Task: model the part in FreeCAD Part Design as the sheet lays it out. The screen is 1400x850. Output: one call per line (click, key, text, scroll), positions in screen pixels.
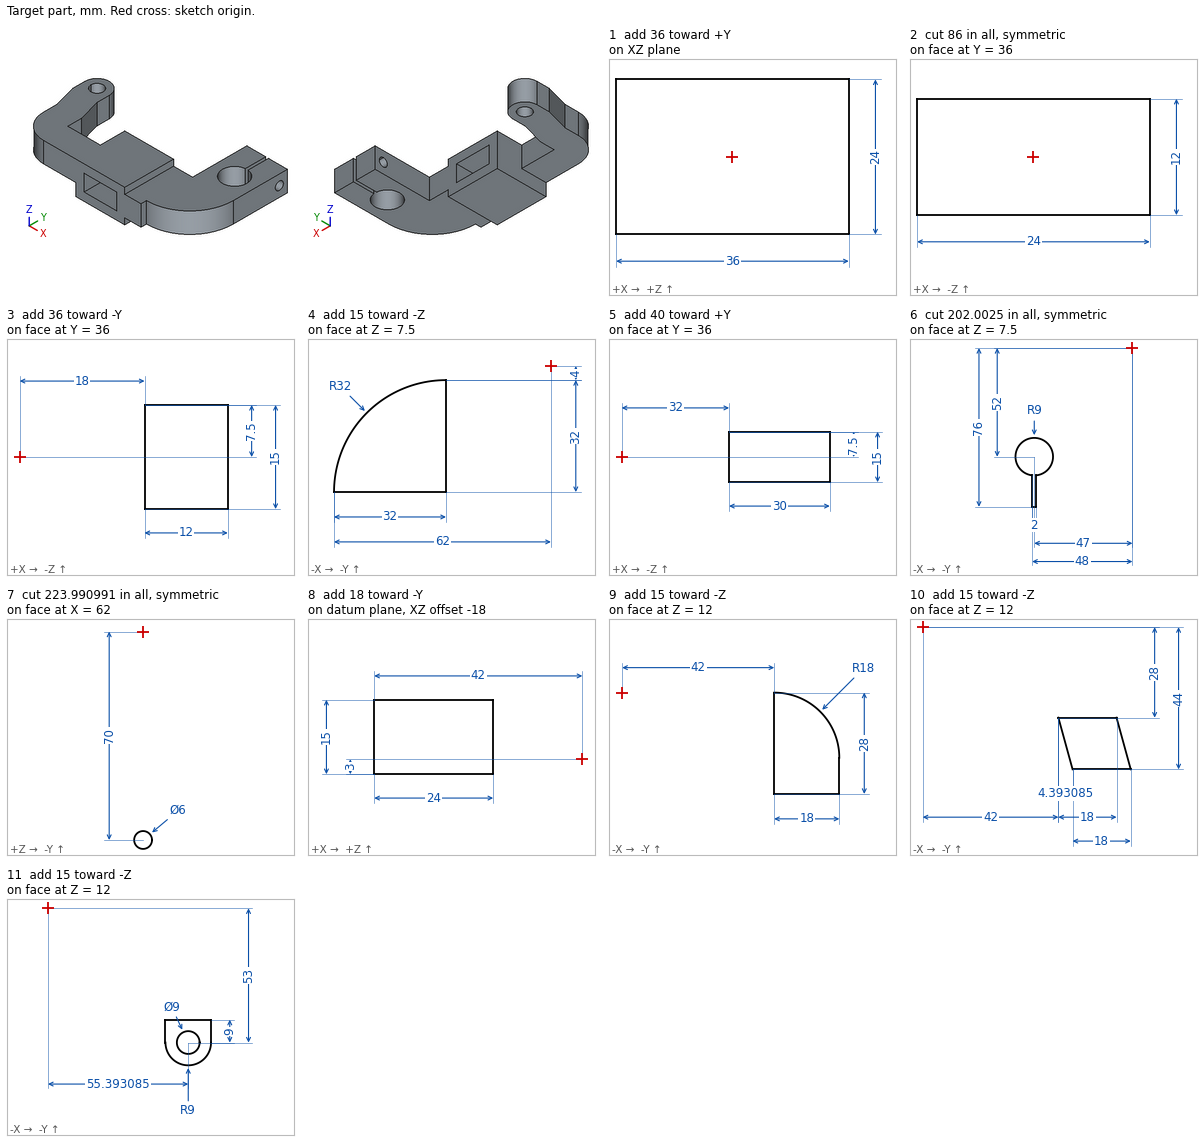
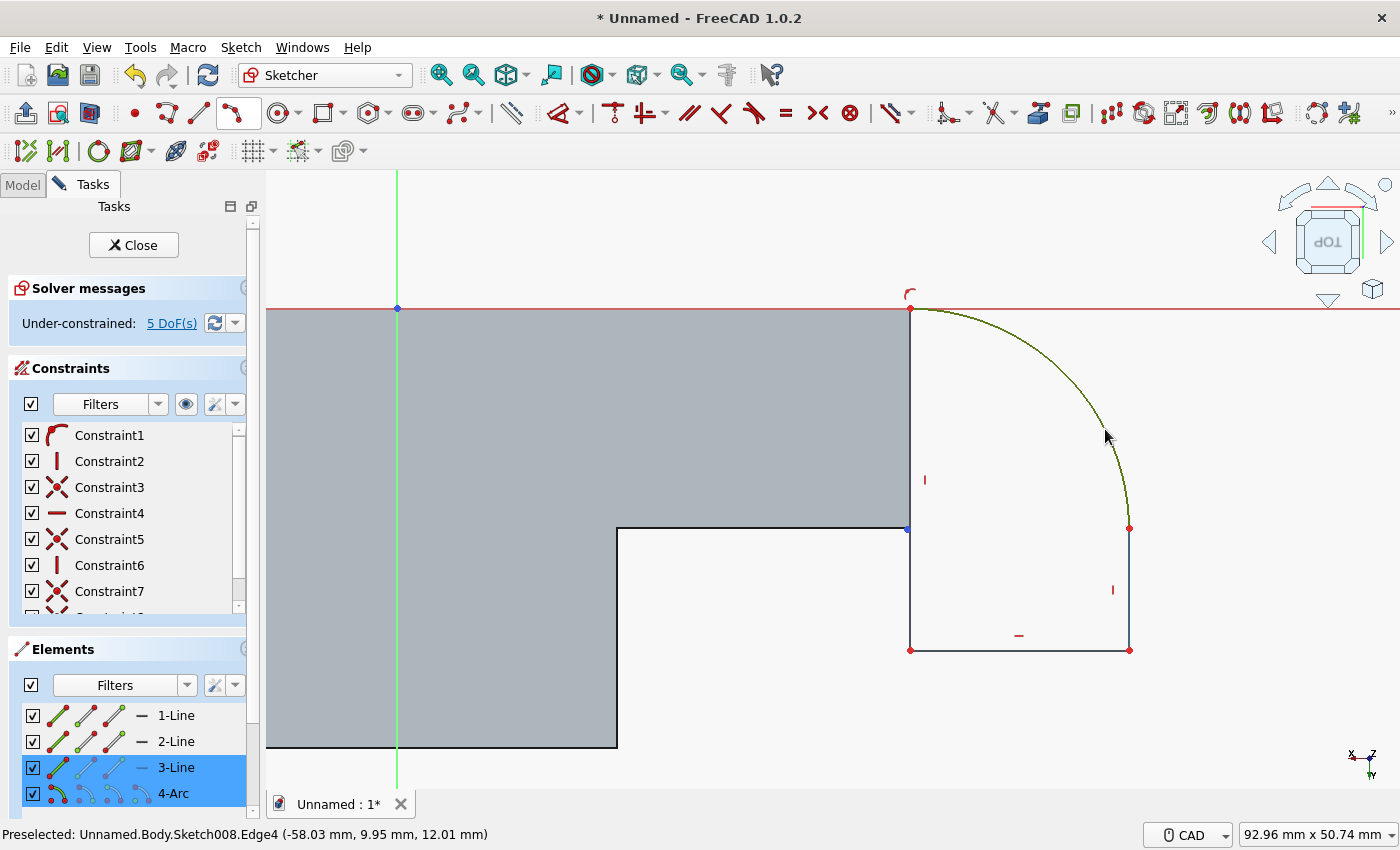
key(t)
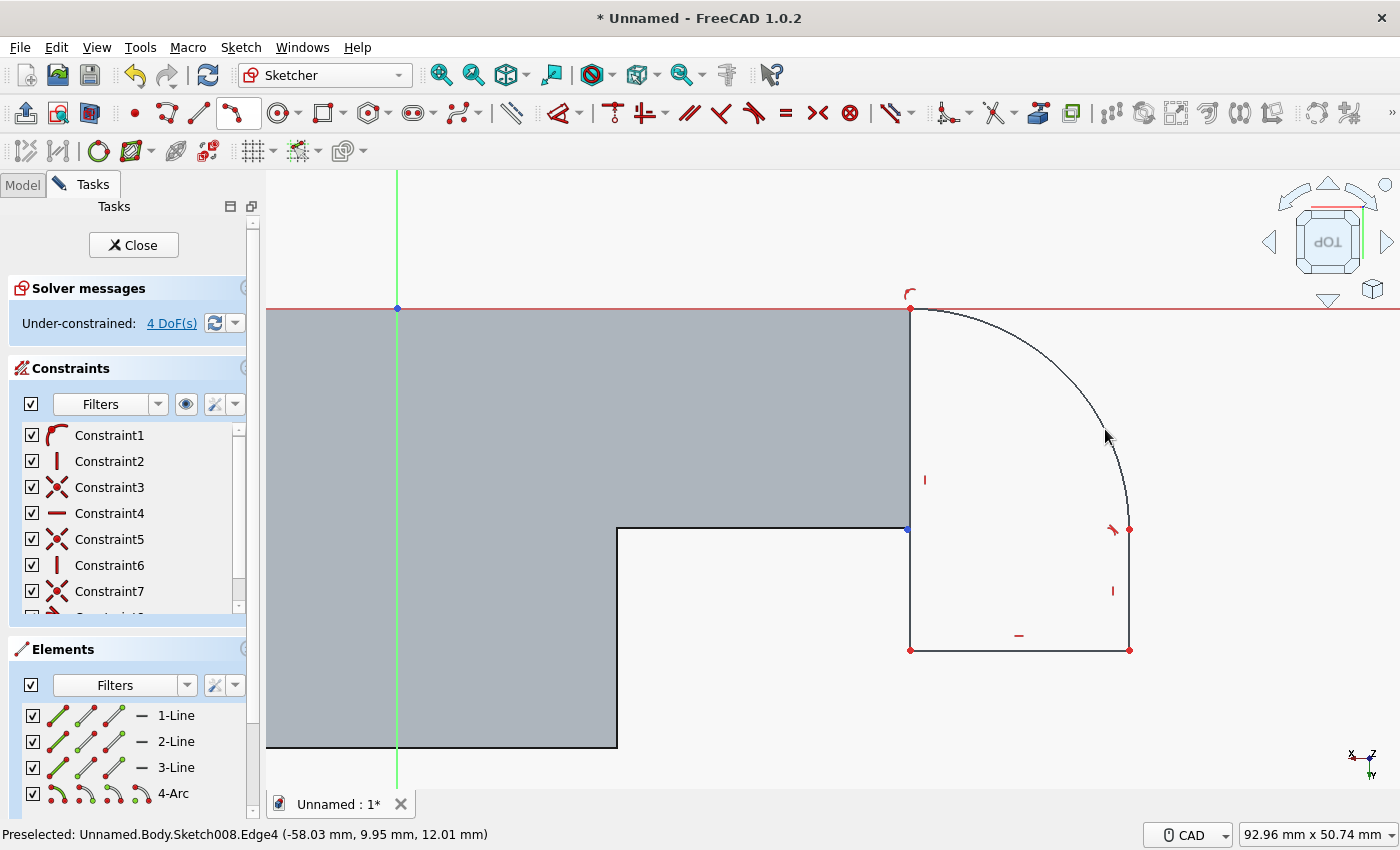
key(d)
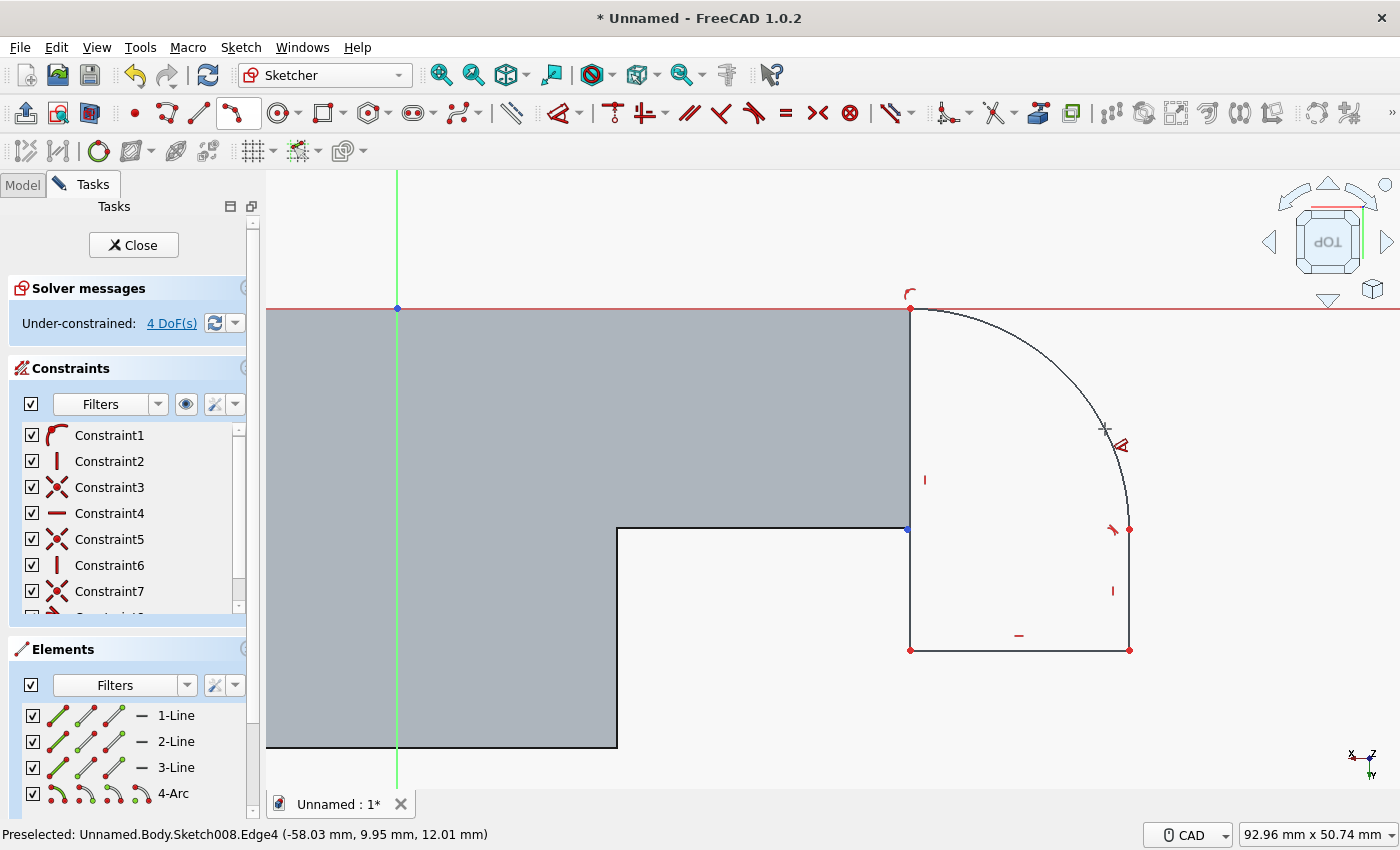
click(1105, 430)
click(1134, 416)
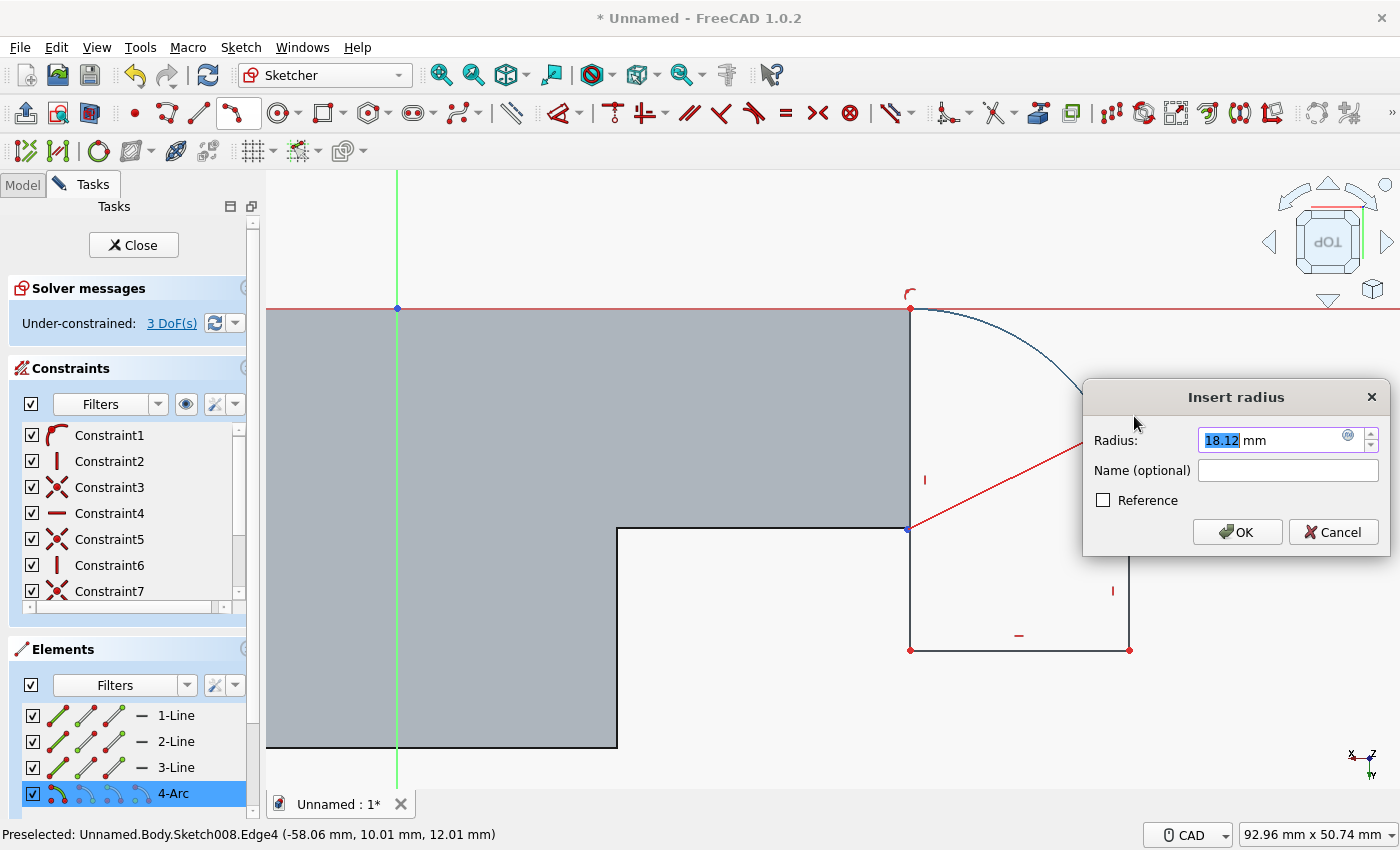
text(18)
key(Return)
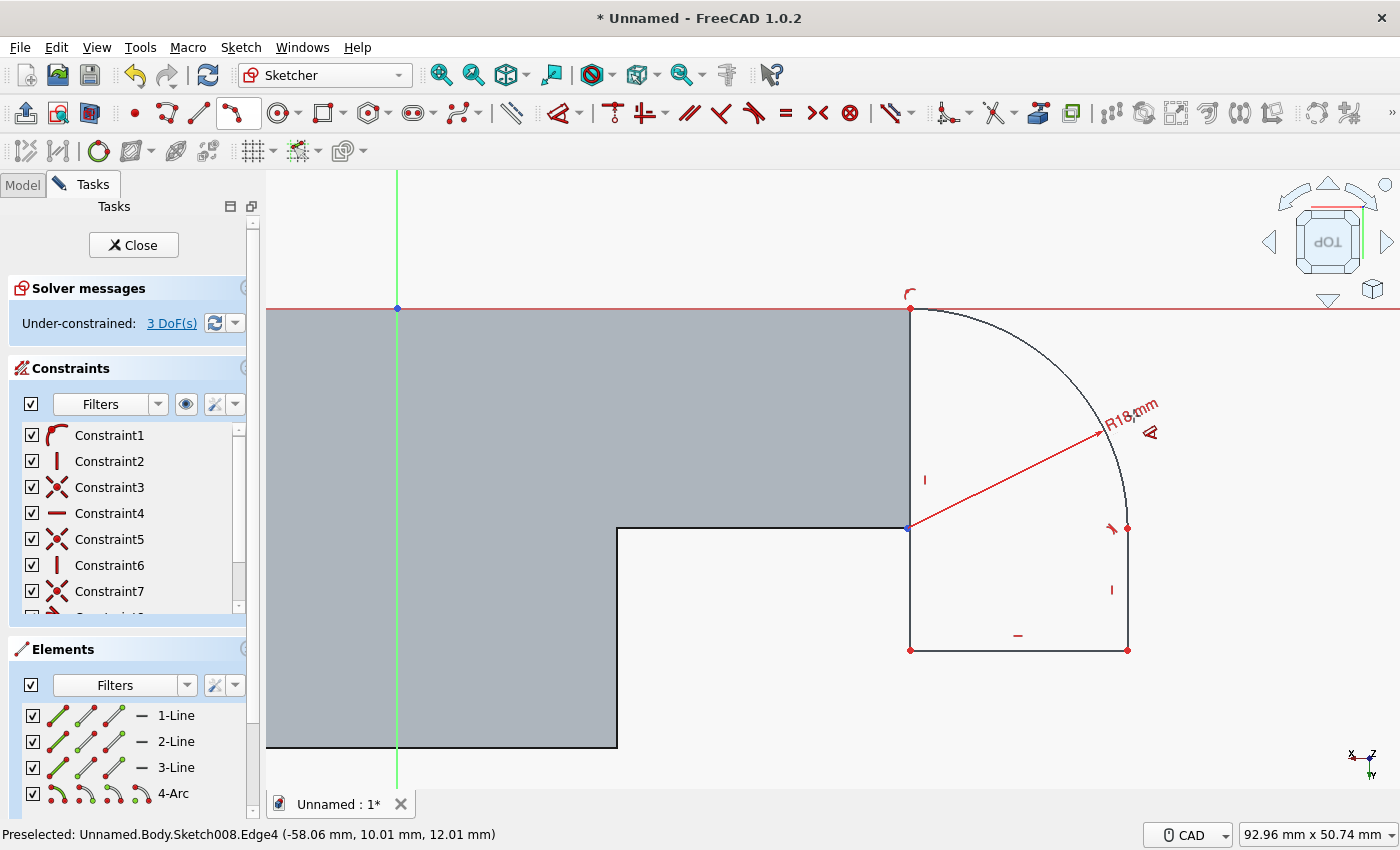
click(910, 411)
click(944, 480)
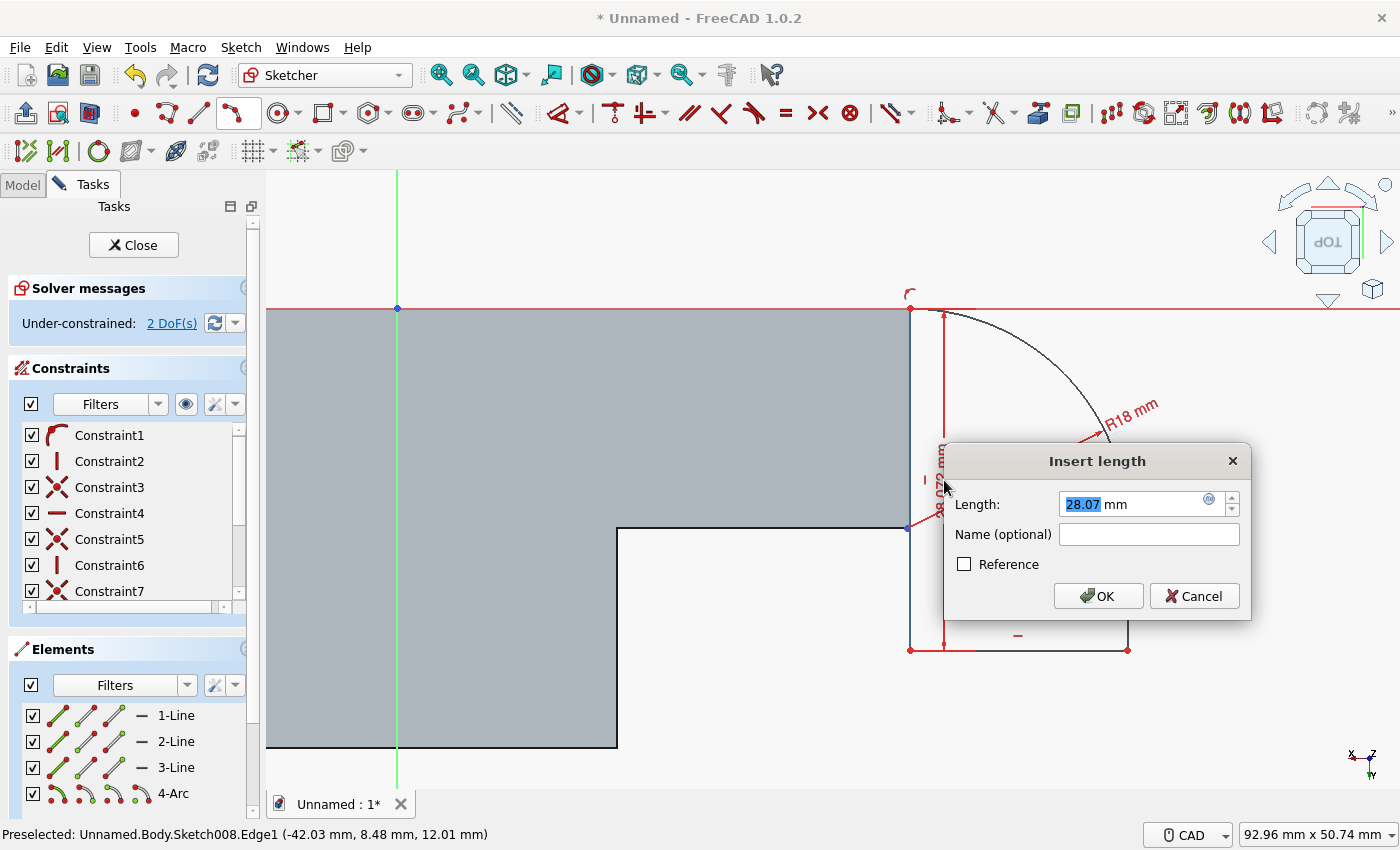
text(28)
key(Return)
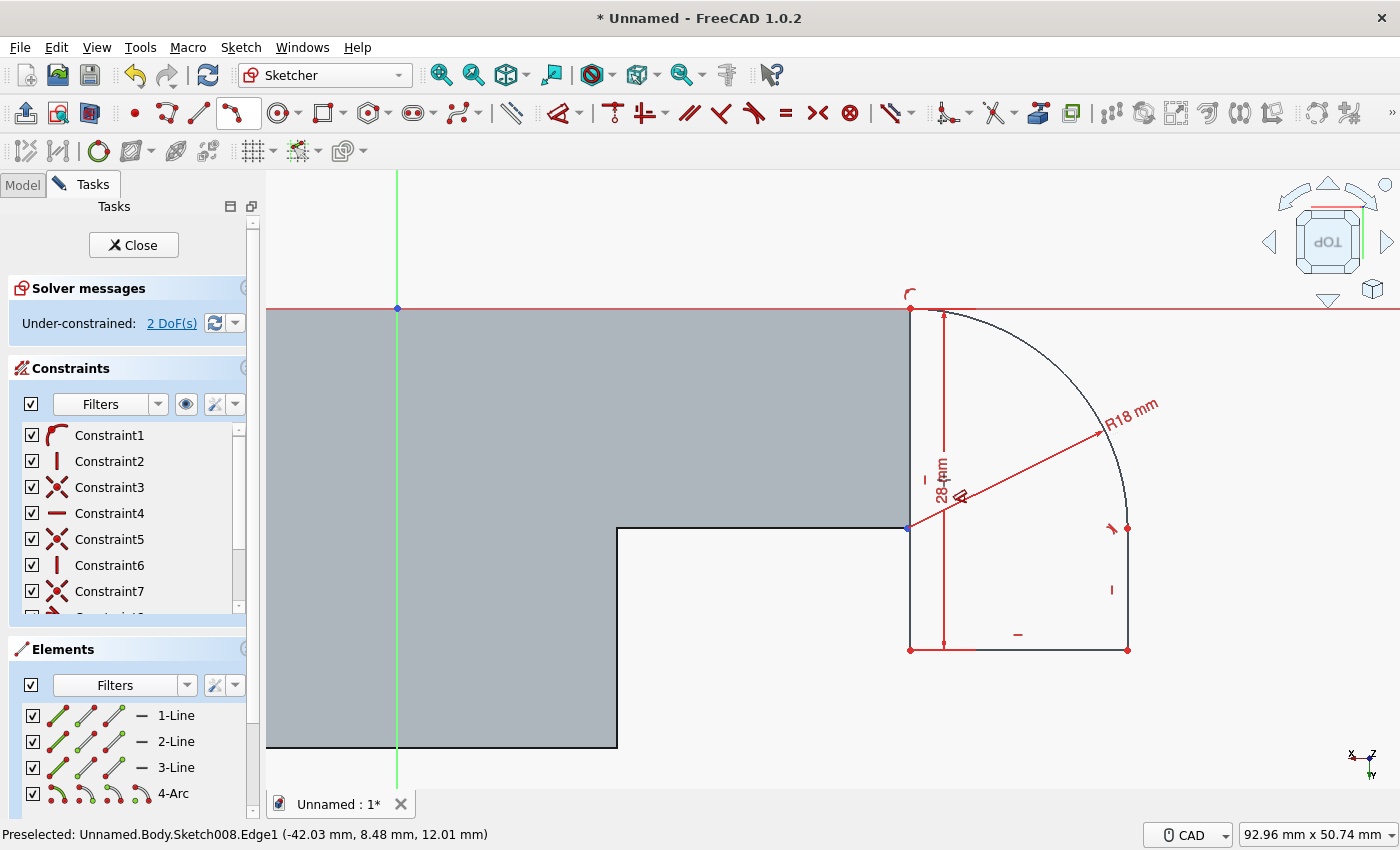
click(975, 650)
click(1019, 684)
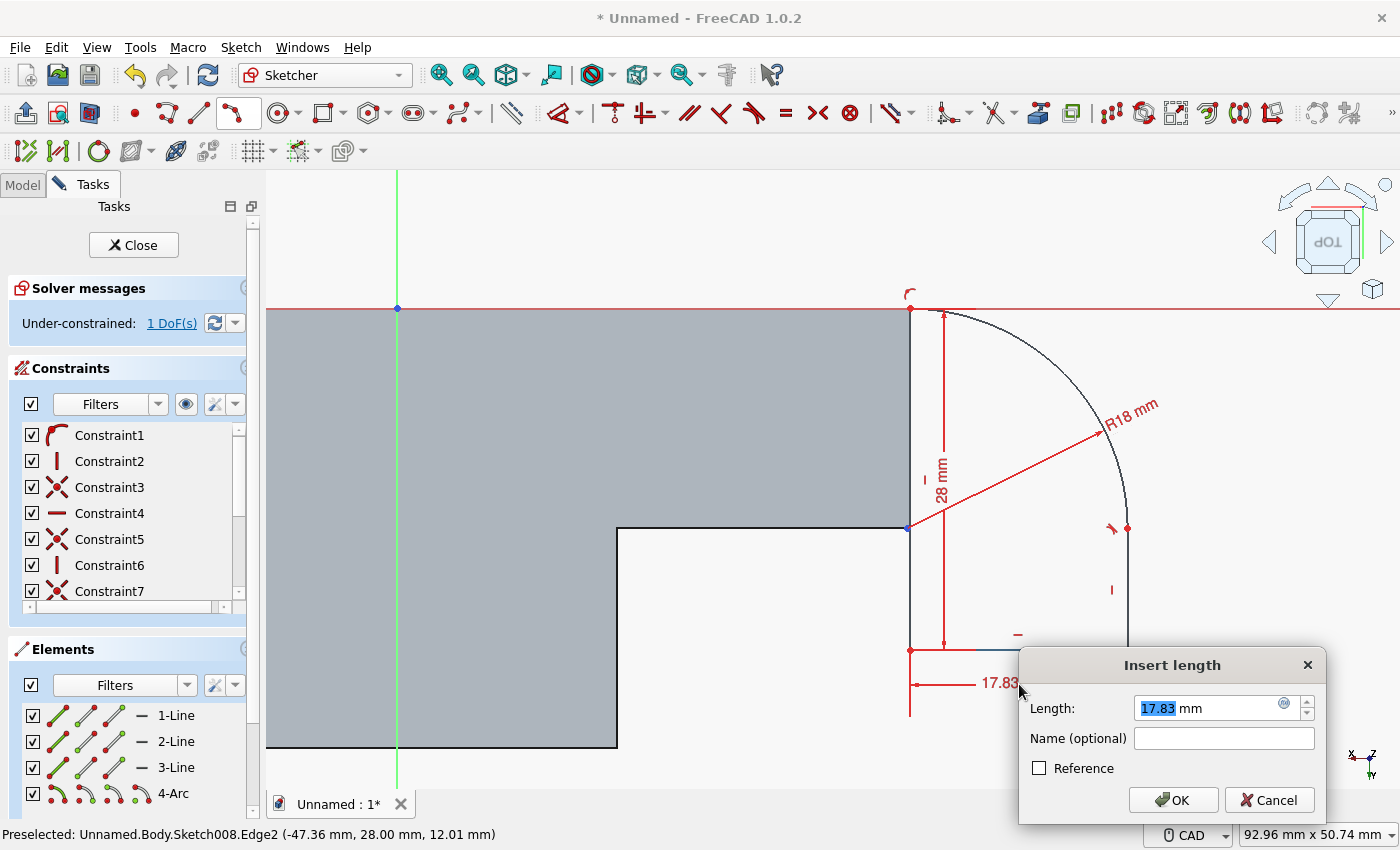
text(18)
key(Return)